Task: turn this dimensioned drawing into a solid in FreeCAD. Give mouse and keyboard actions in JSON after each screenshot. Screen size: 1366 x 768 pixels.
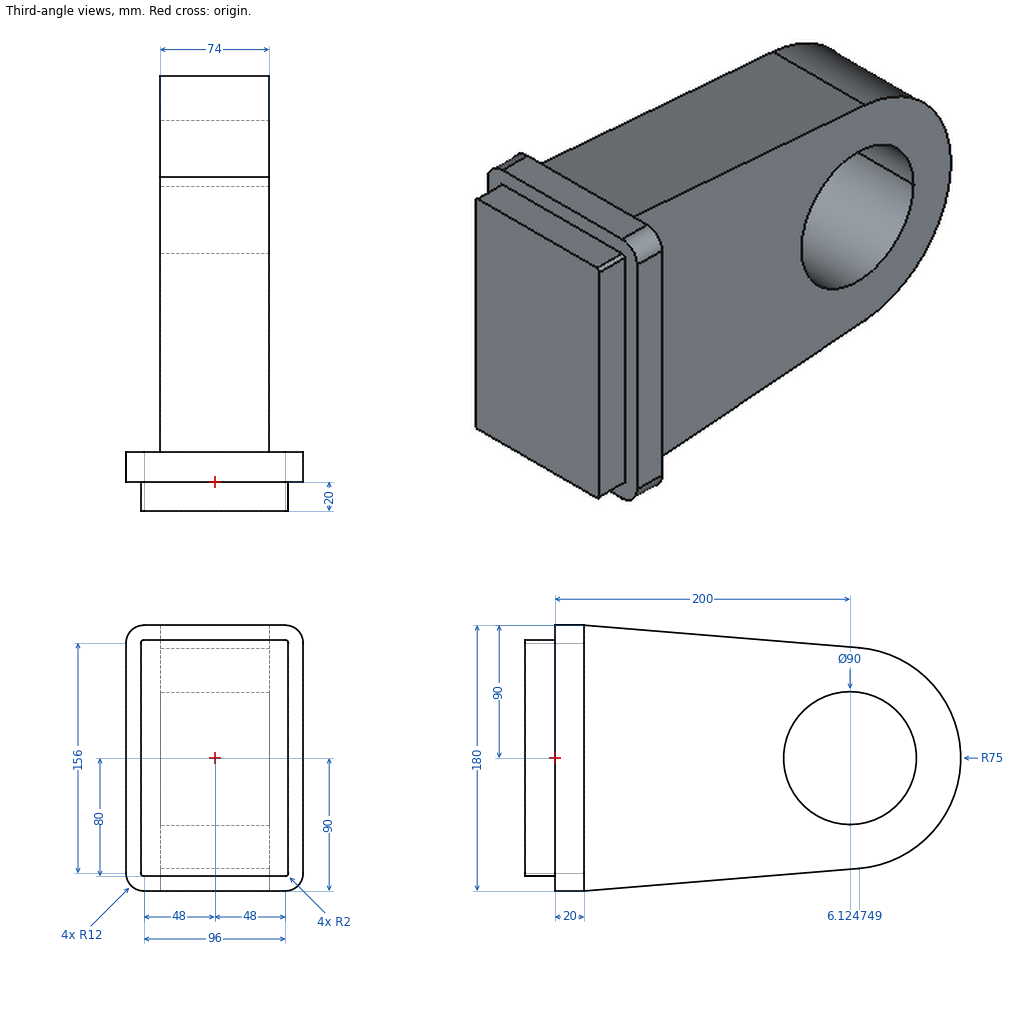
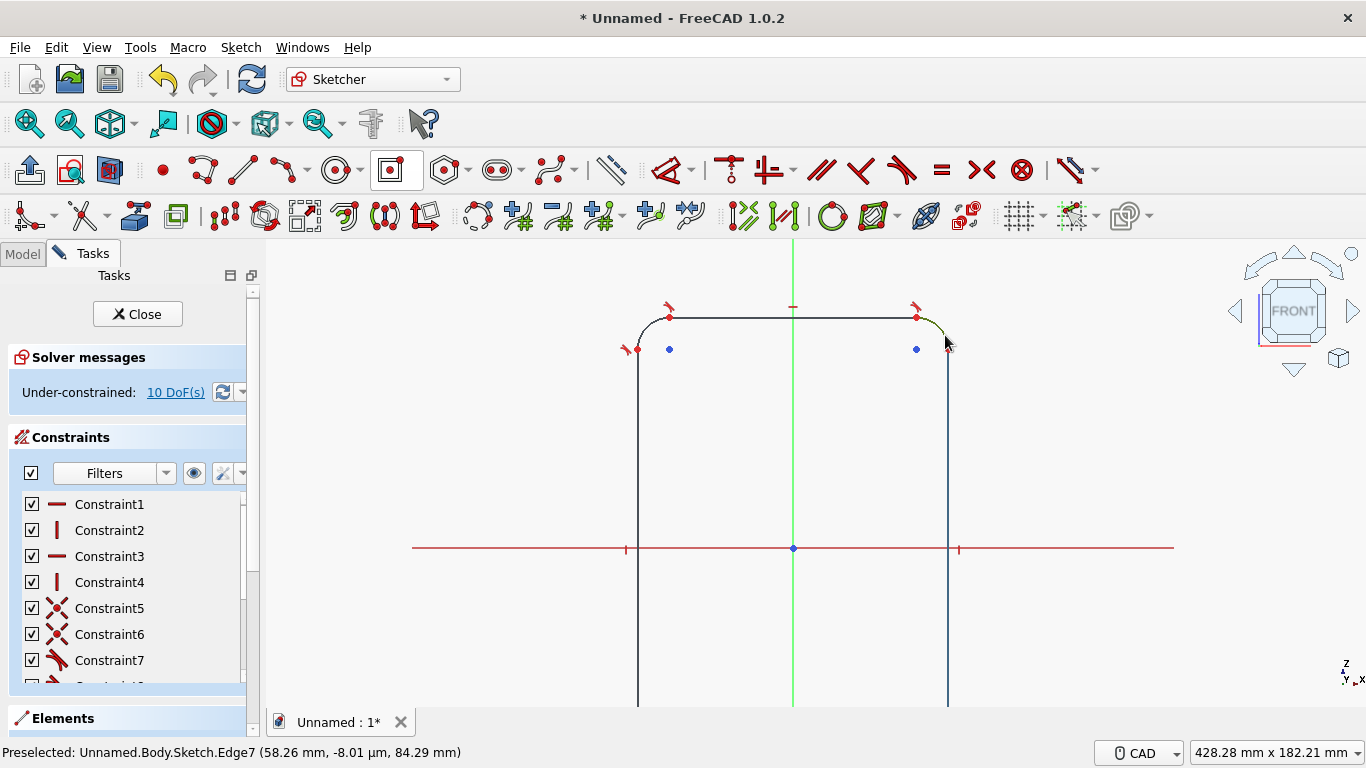
{"action": "key", "text": "t"}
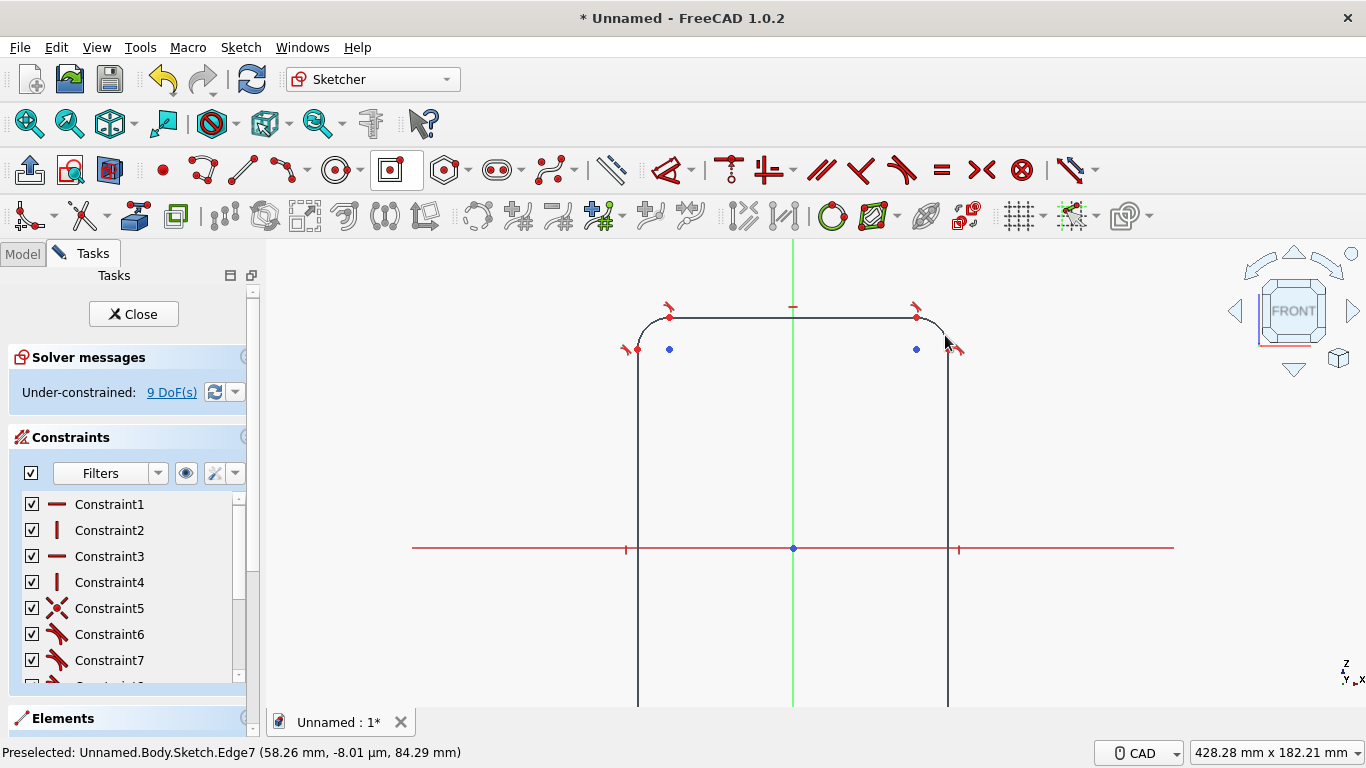
{"action": "left_click", "coordinate": [948, 470]}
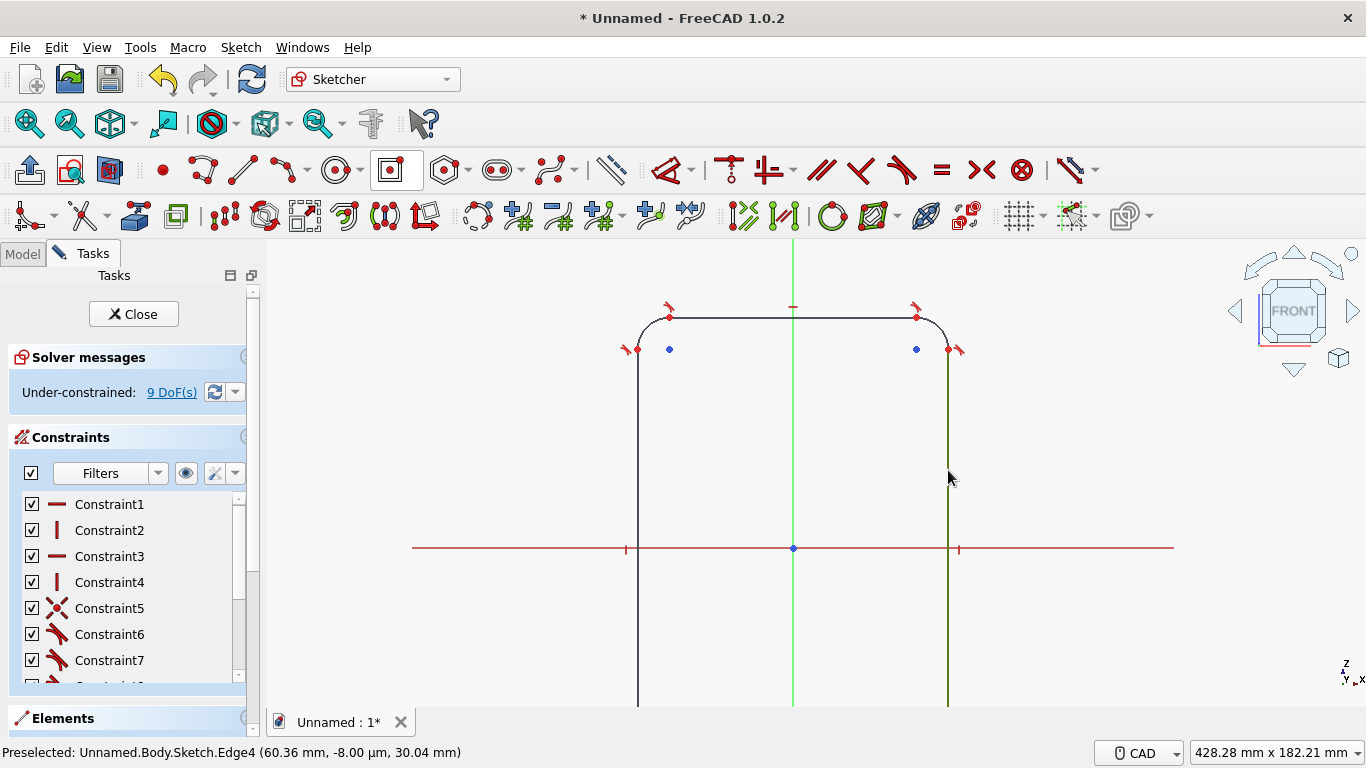
{"action": "scroll", "coordinate": [655, 320], "scroll_direction": "down", "scroll_amount": 2}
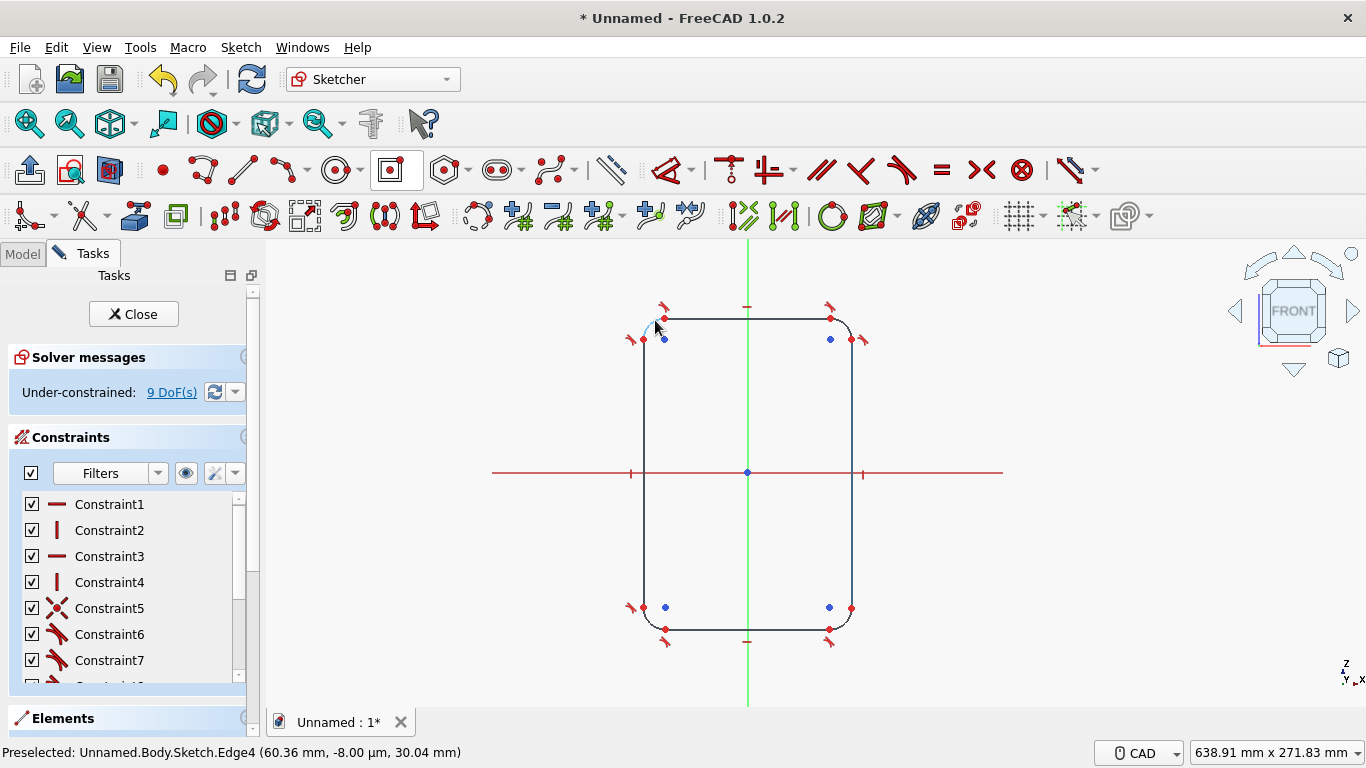
{"action": "scroll", "coordinate": [840, 627], "scroll_direction": "up", "scroll_amount": 2}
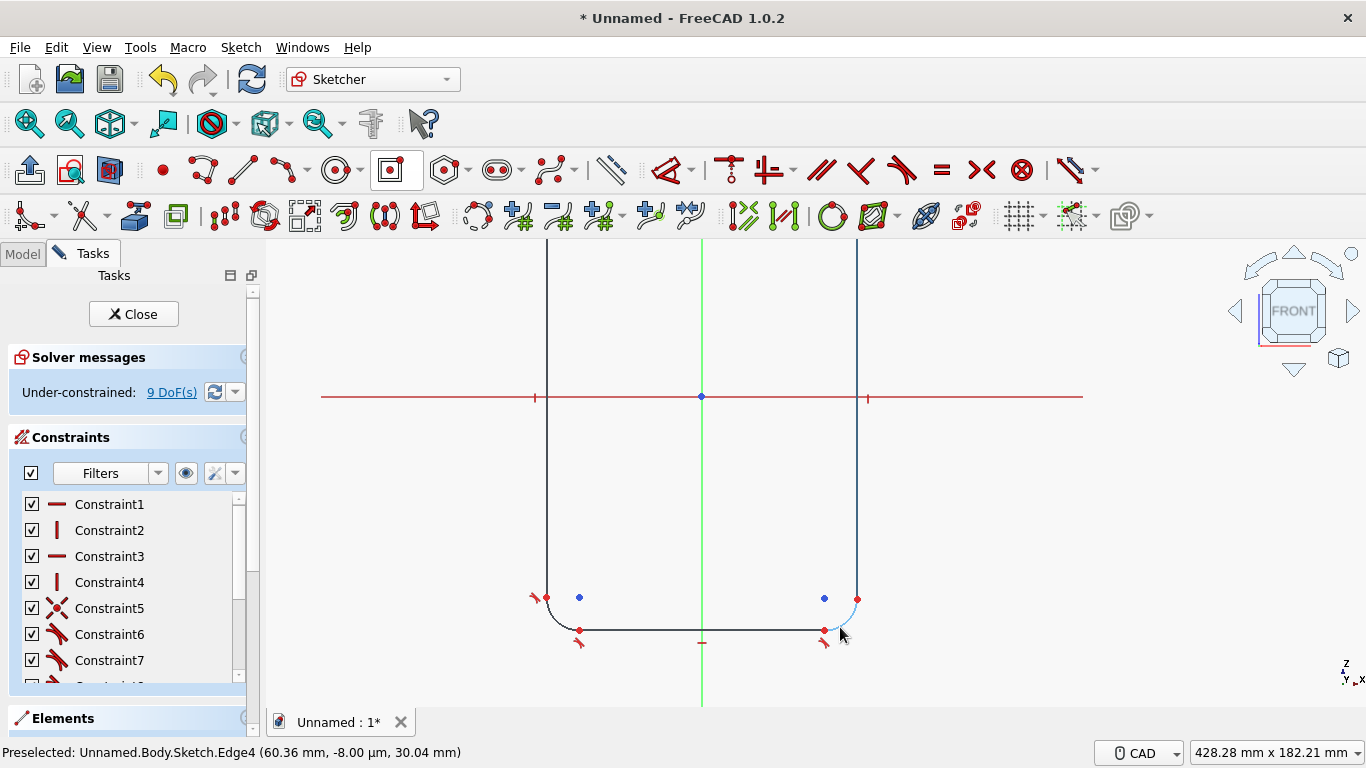
{"action": "left_click", "coordinate": [839, 627]}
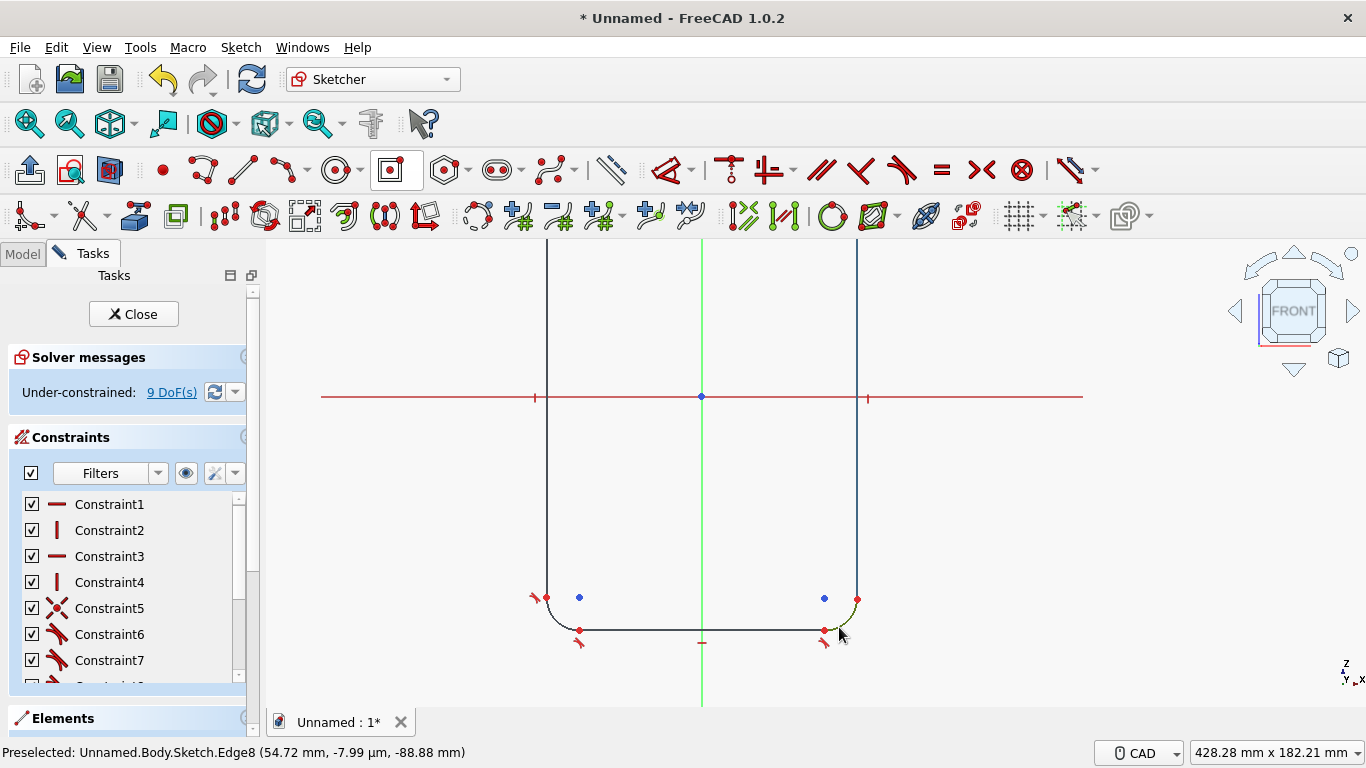
{"action": "key", "text": "t"}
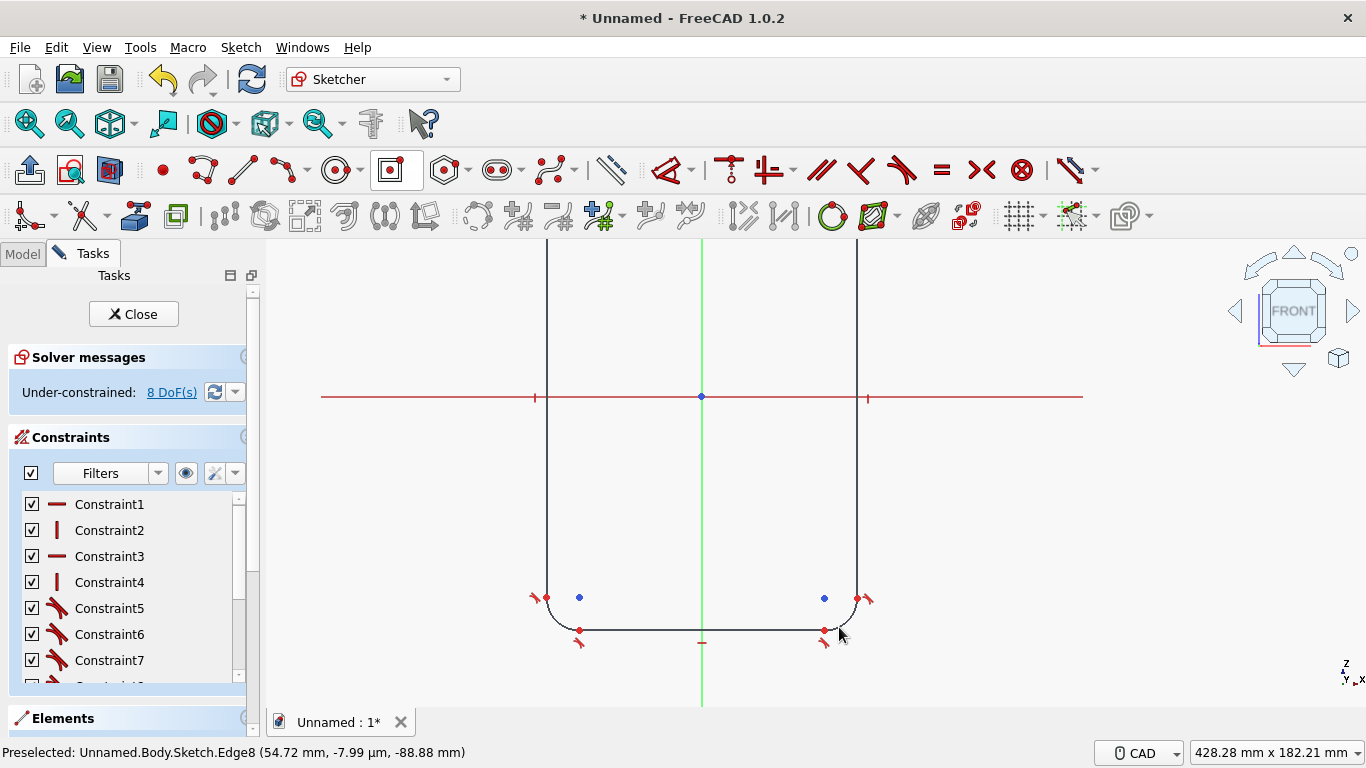
{"action": "left_click", "coordinate": [550, 613]}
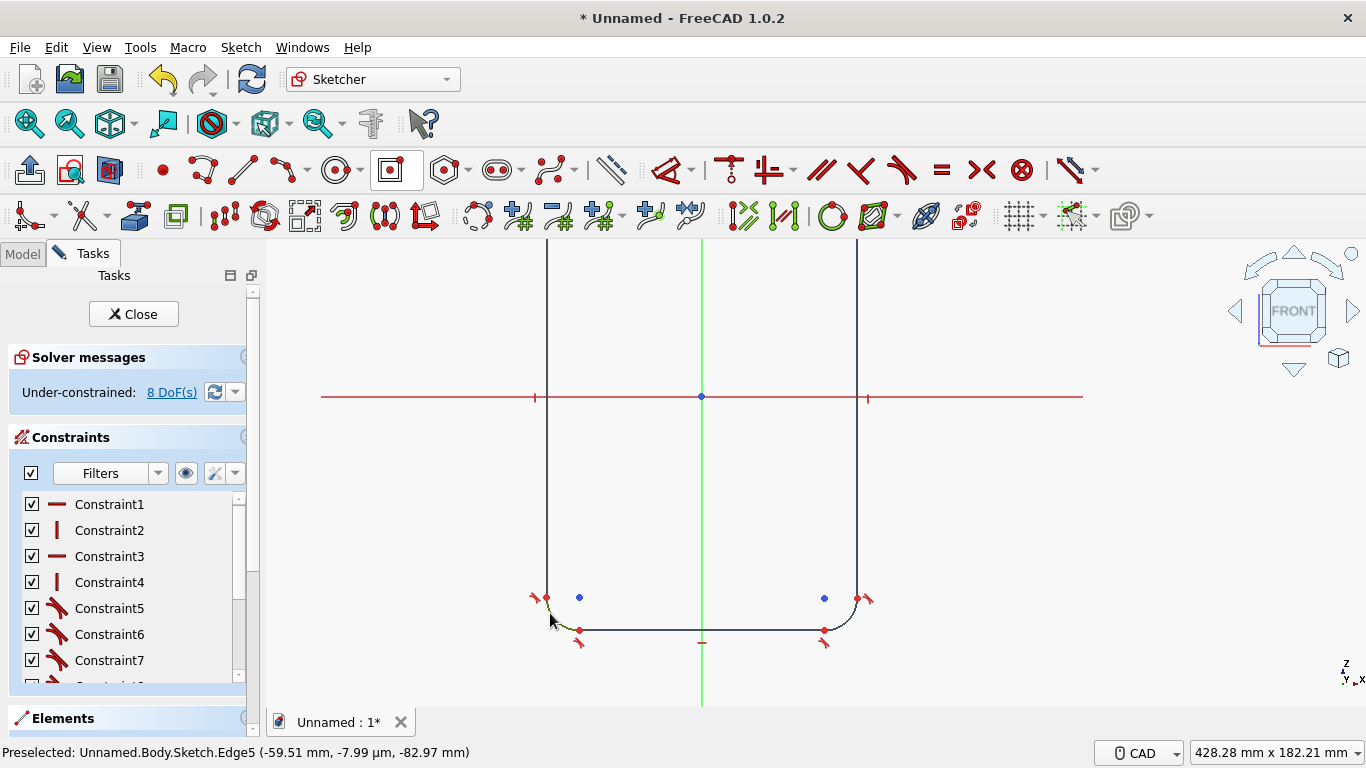
{"action": "scroll", "coordinate": [840, 628], "scroll_direction": "down", "scroll_amount": 2}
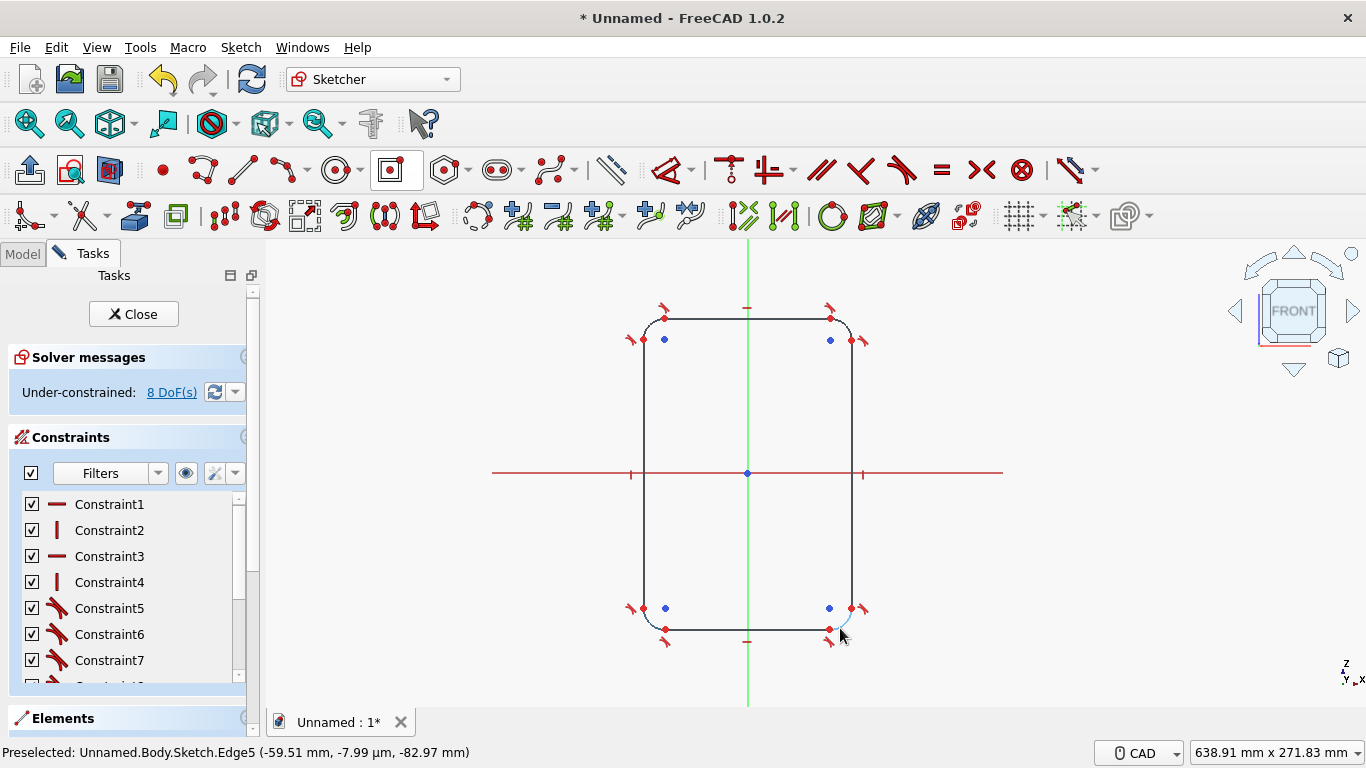
{"action": "scroll", "coordinate": [655, 321], "scroll_direction": "up", "scroll_amount": 2}